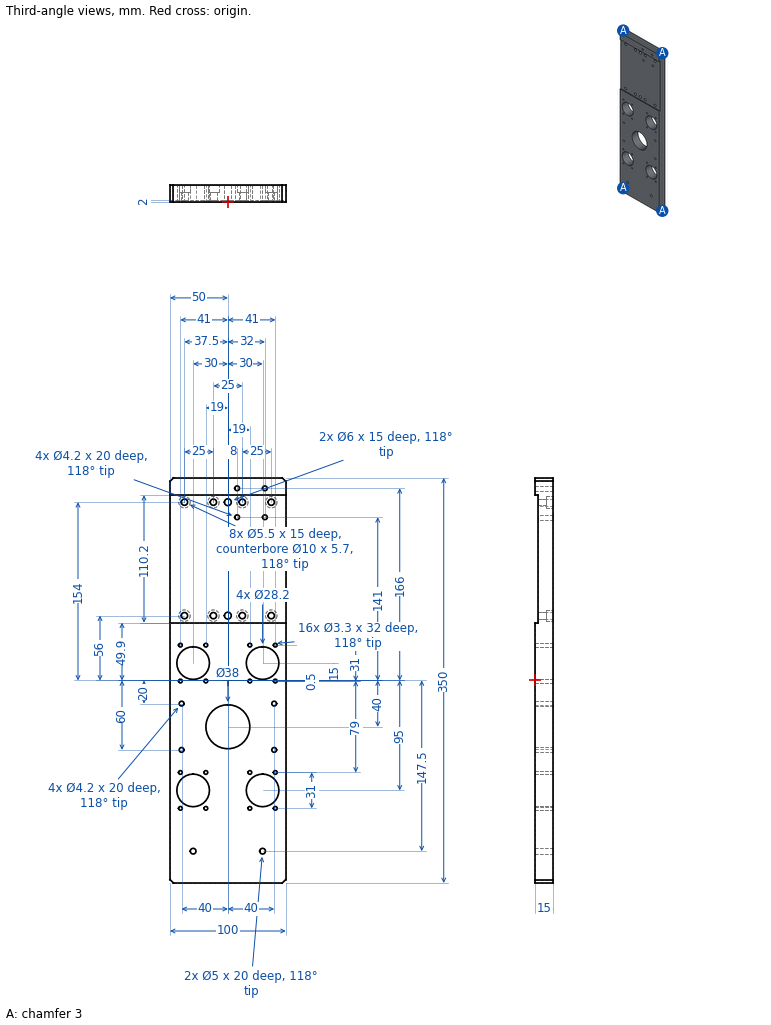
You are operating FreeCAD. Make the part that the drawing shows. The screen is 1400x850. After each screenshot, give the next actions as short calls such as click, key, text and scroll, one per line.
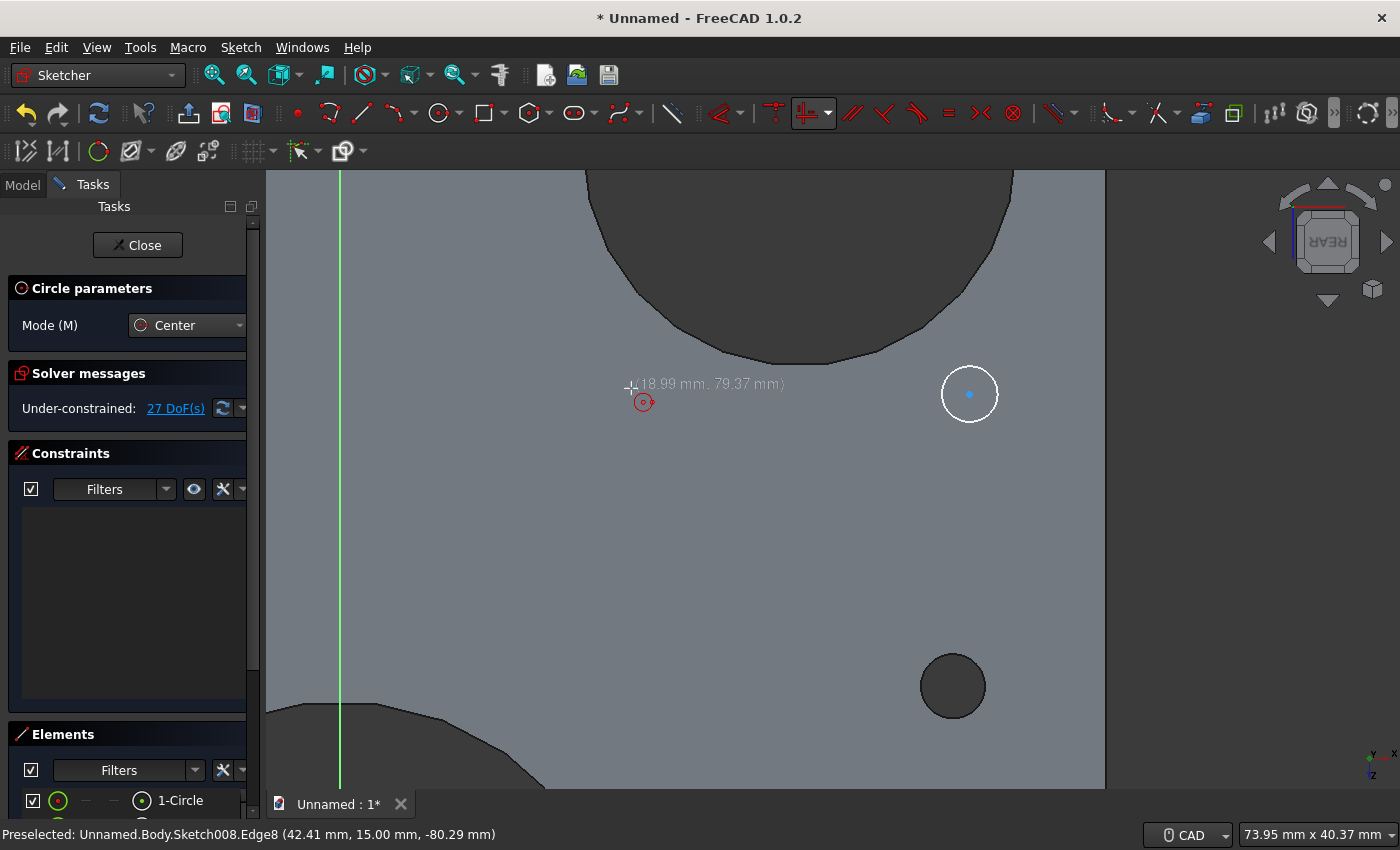
scroll(849, 378, down, 9)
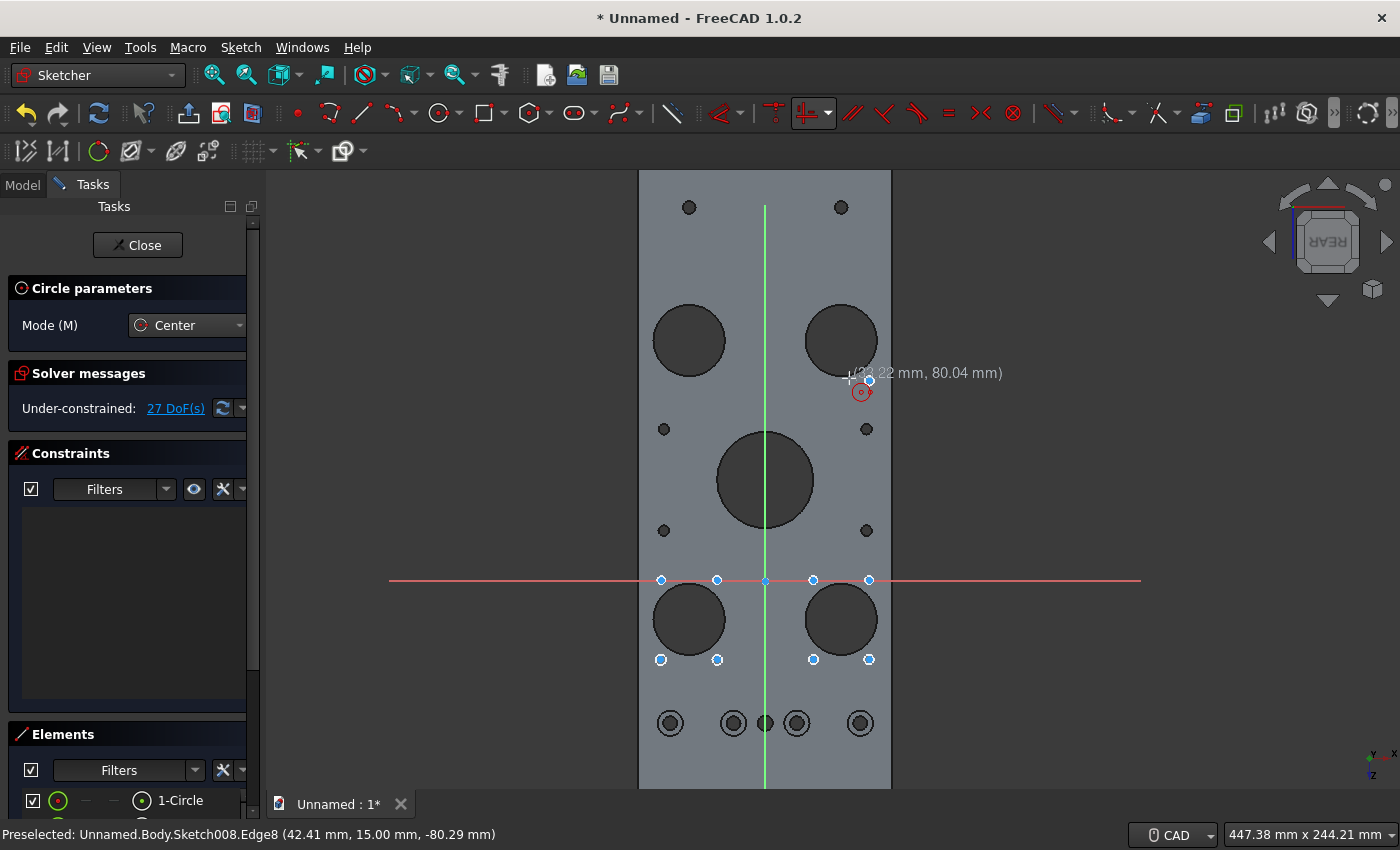
click(813, 380)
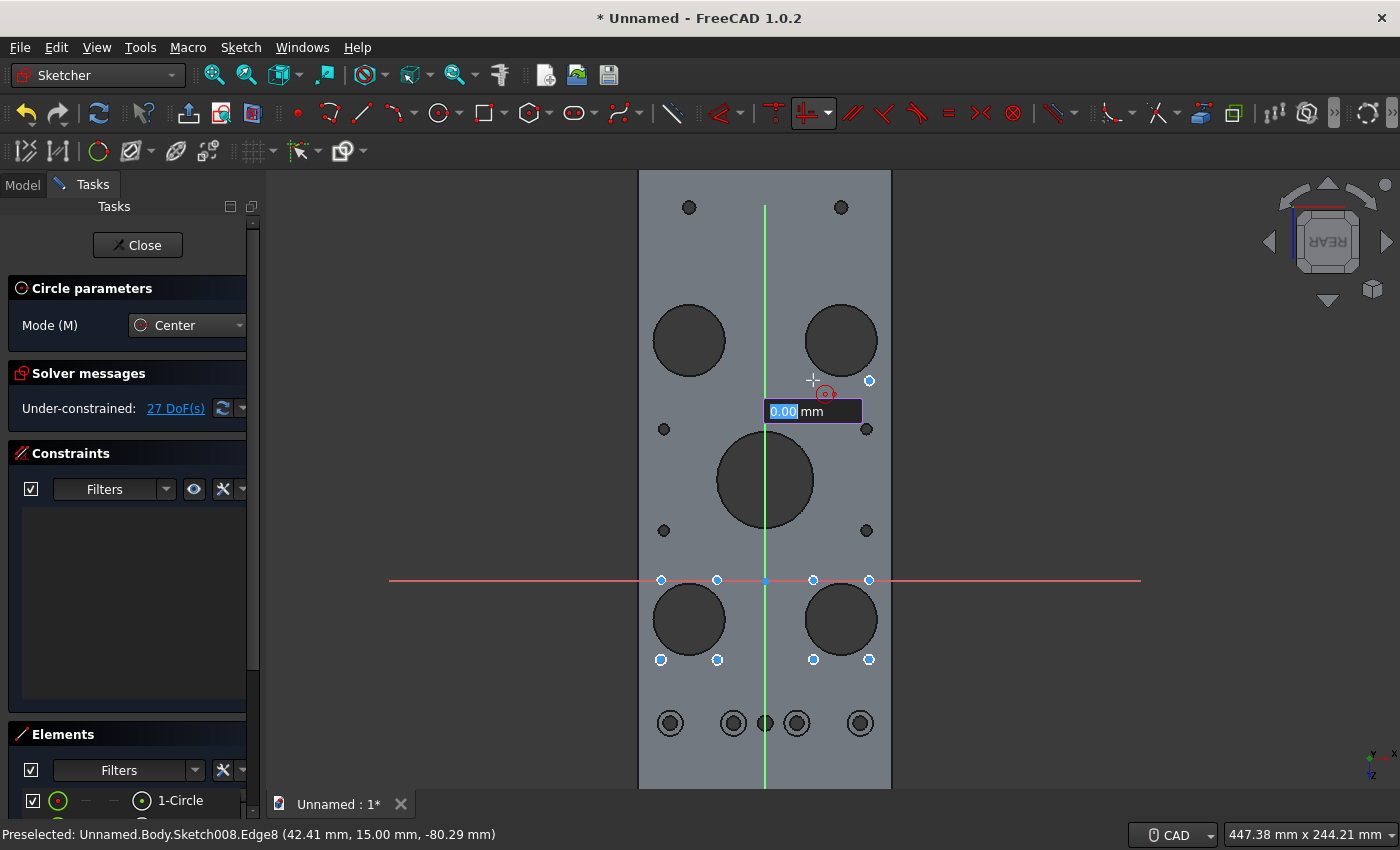
scroll(816, 377, up, 7)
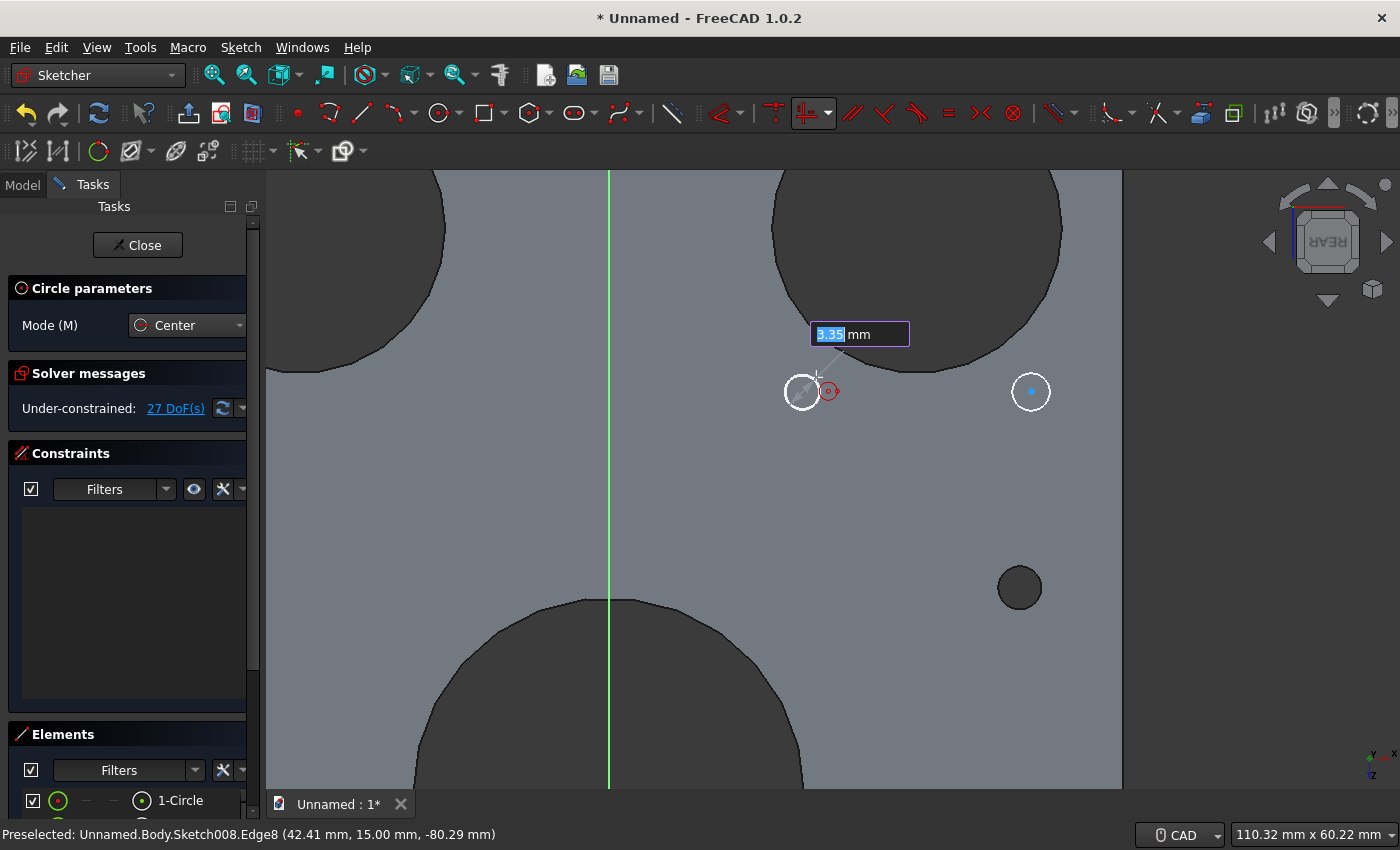
click(816, 375)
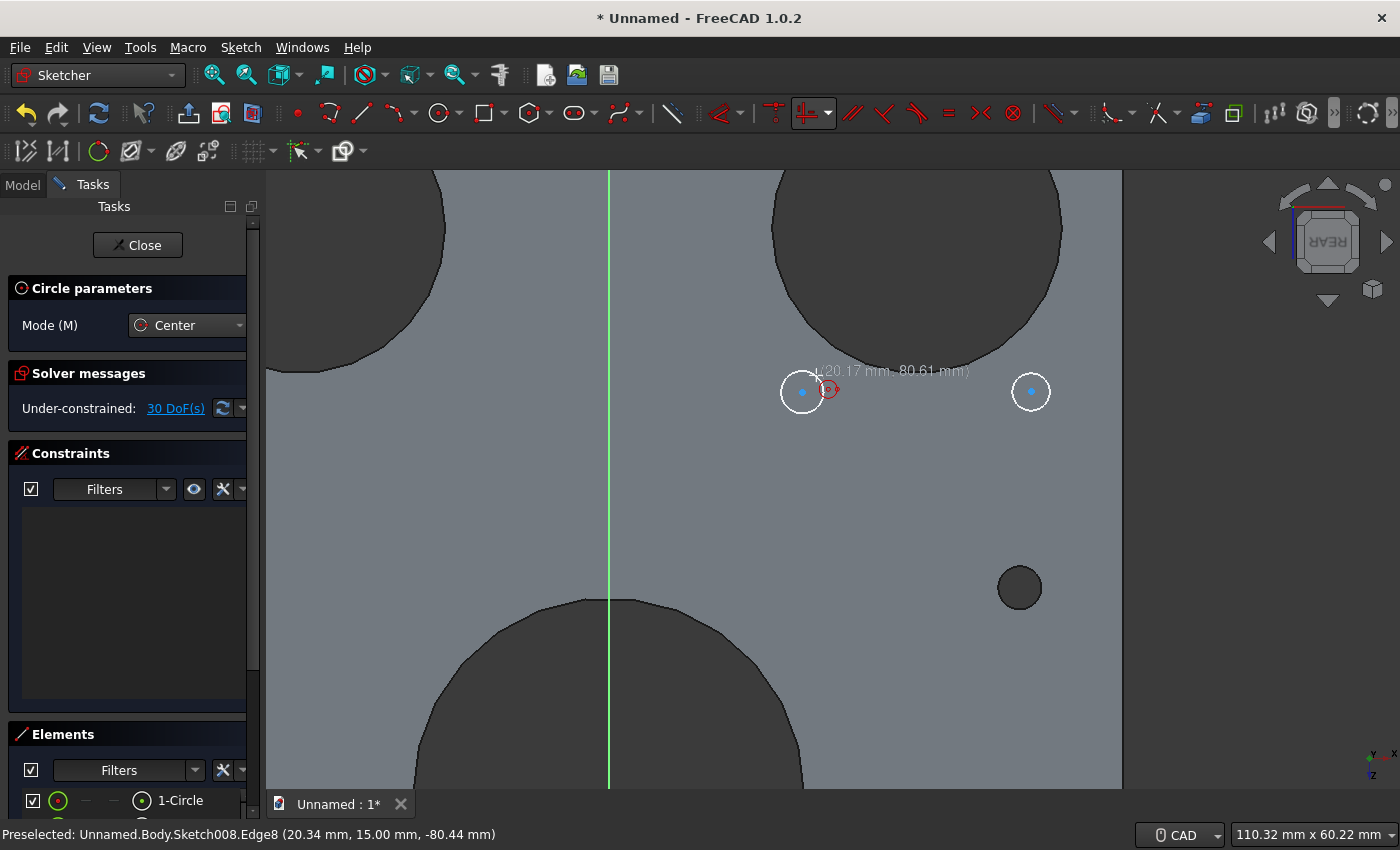
scroll(816, 377, down, 7)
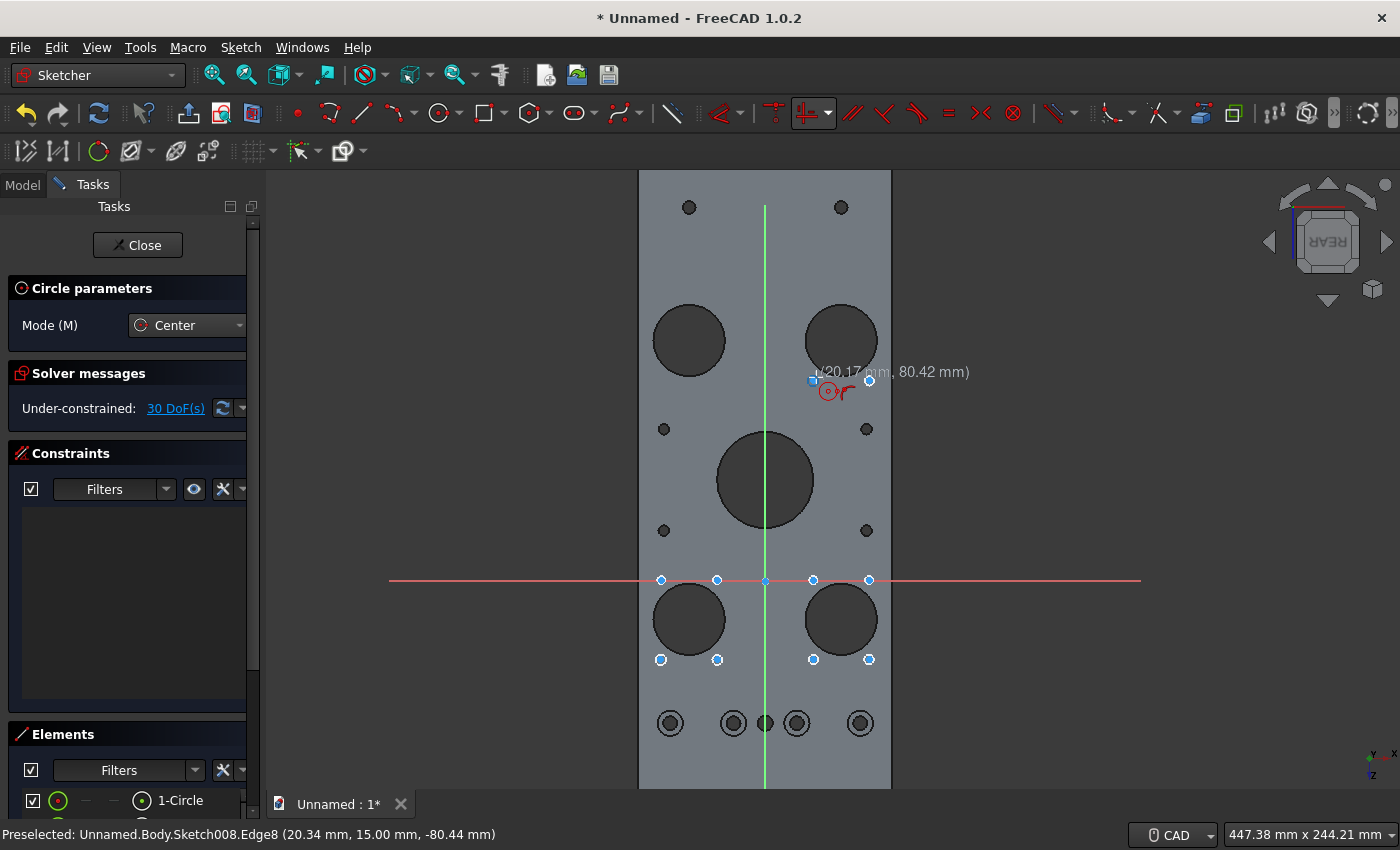
scroll(869, 301, up, 9)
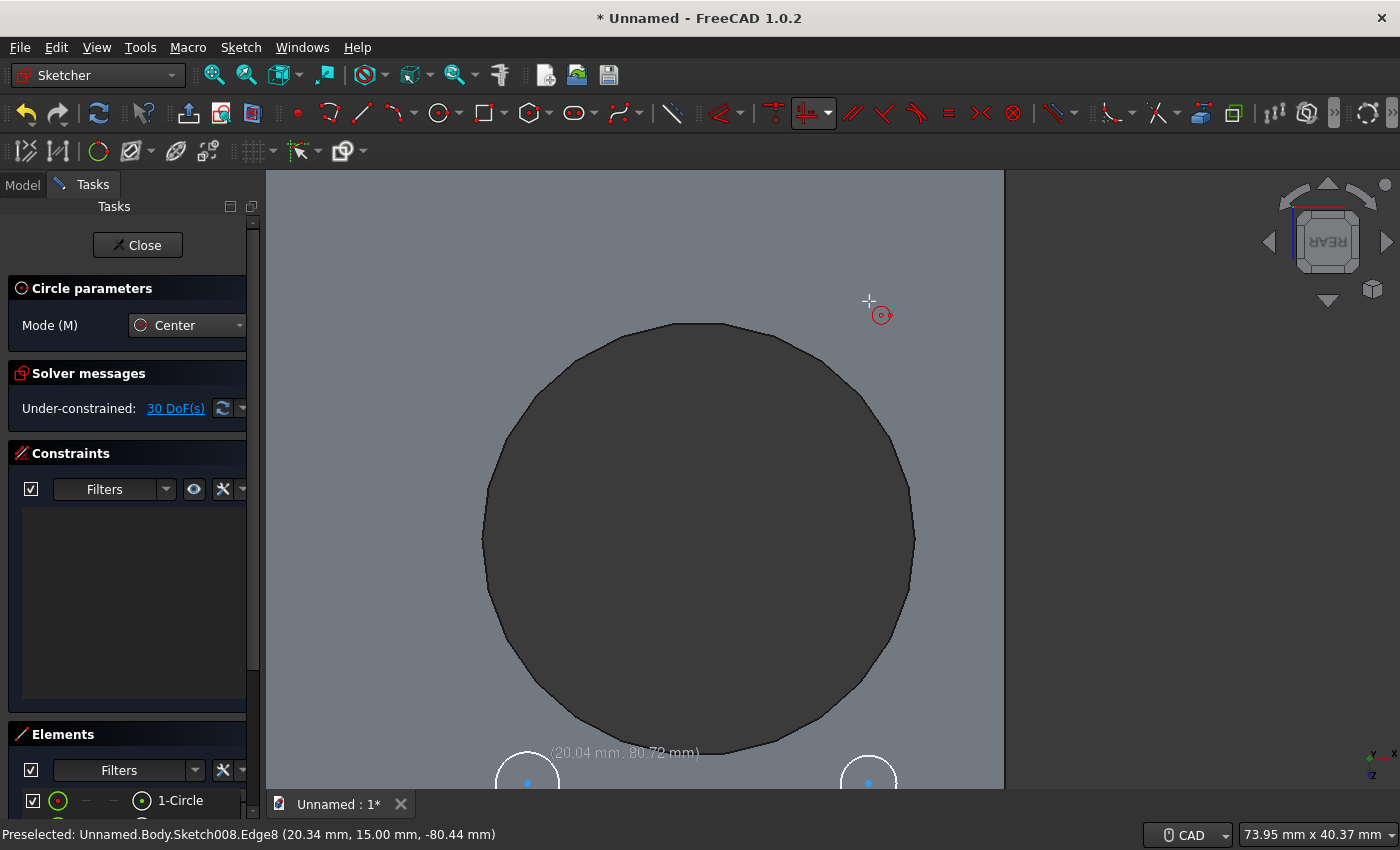
scroll(869, 301, down, 9)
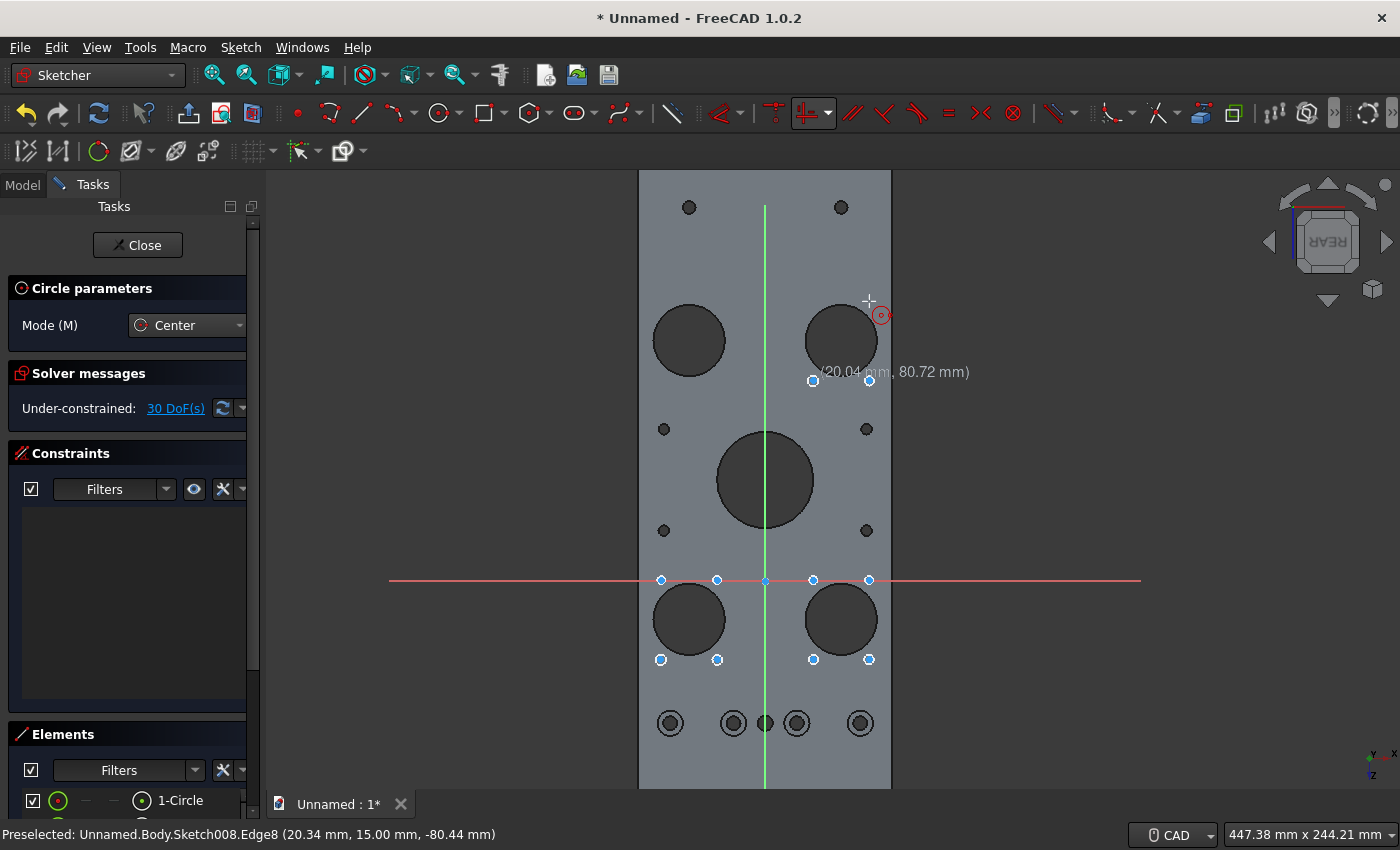
click(869, 301)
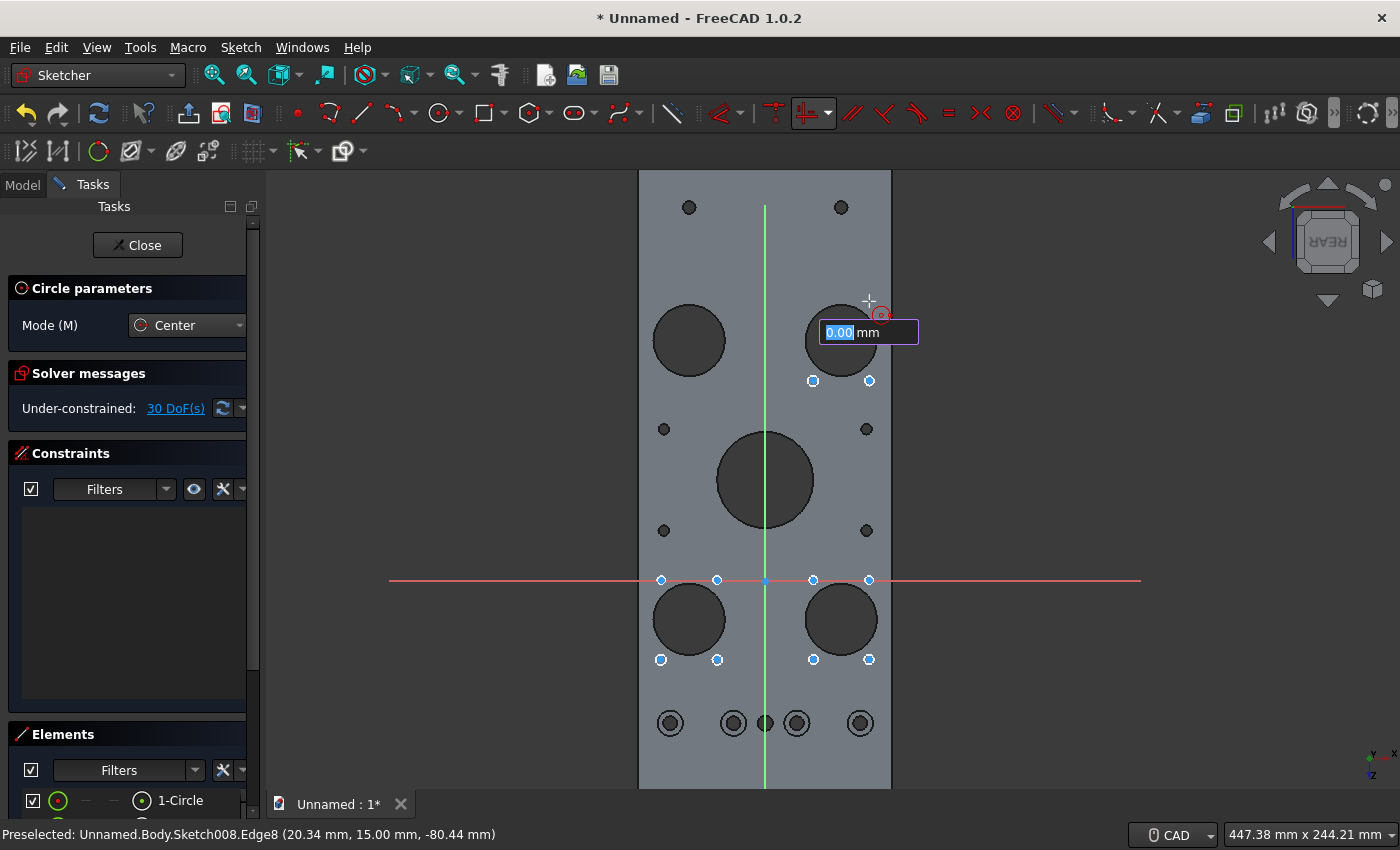
scroll(872, 298, up, 7)